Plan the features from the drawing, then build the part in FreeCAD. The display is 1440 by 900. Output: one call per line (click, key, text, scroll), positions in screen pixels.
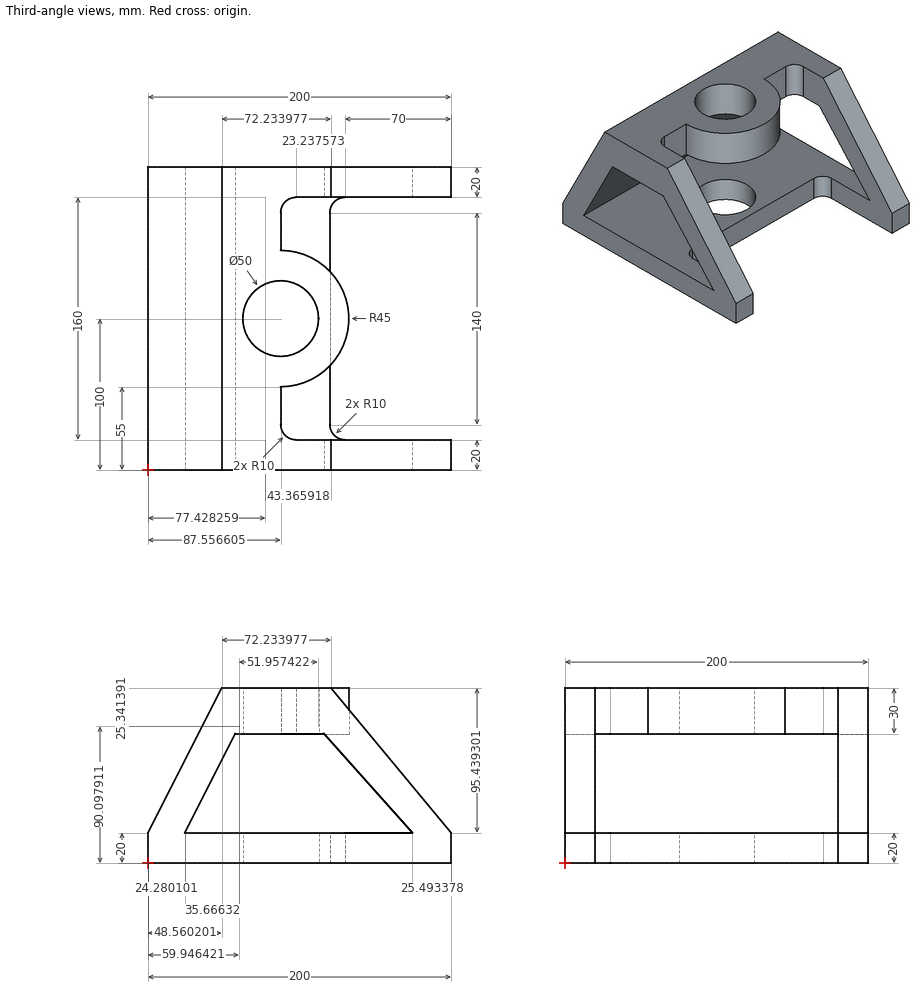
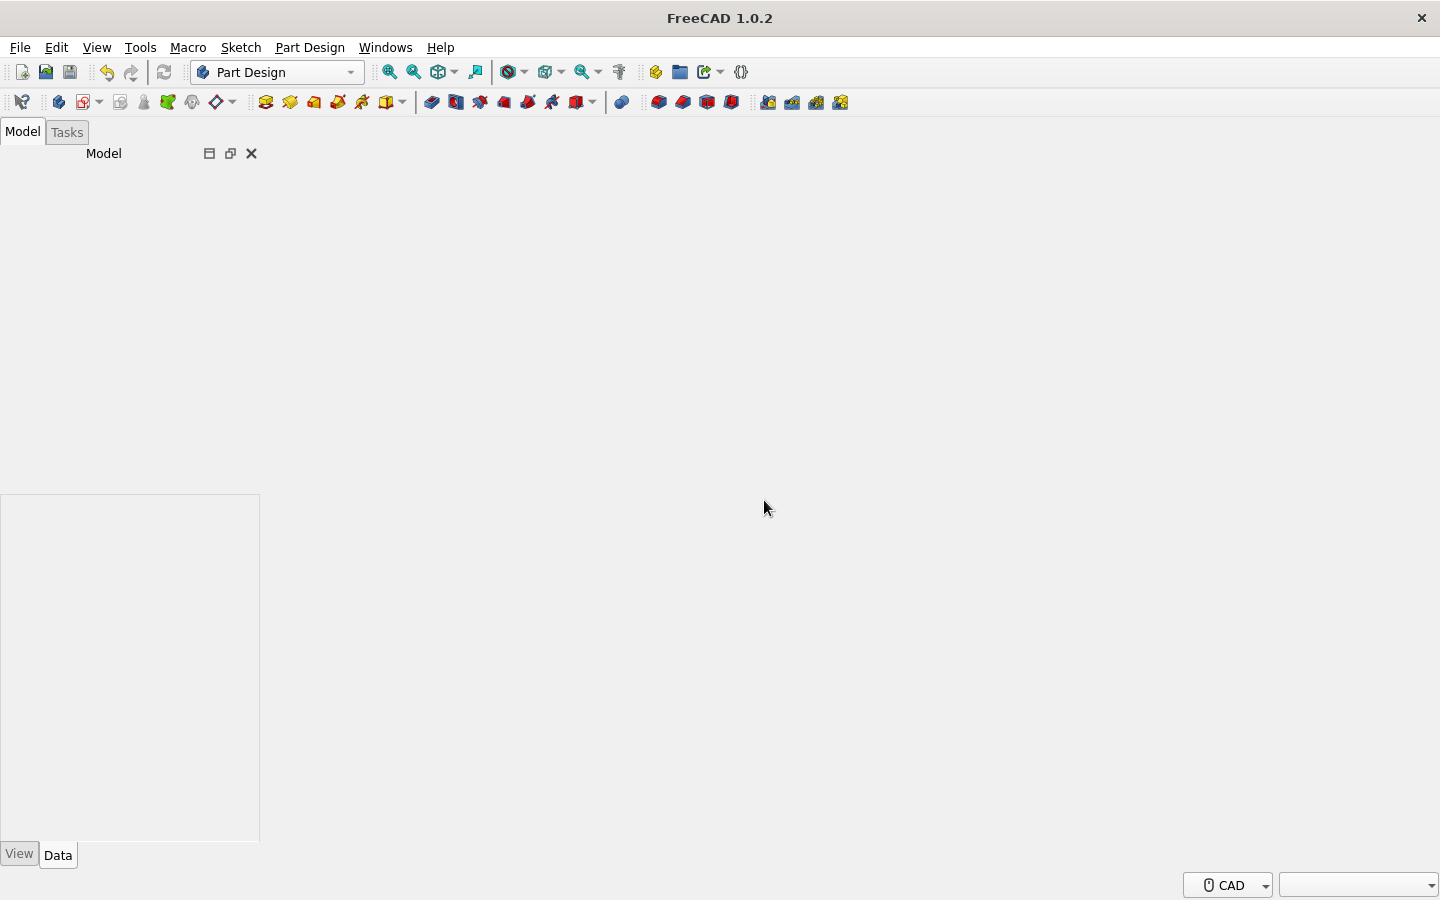
click(22, 72)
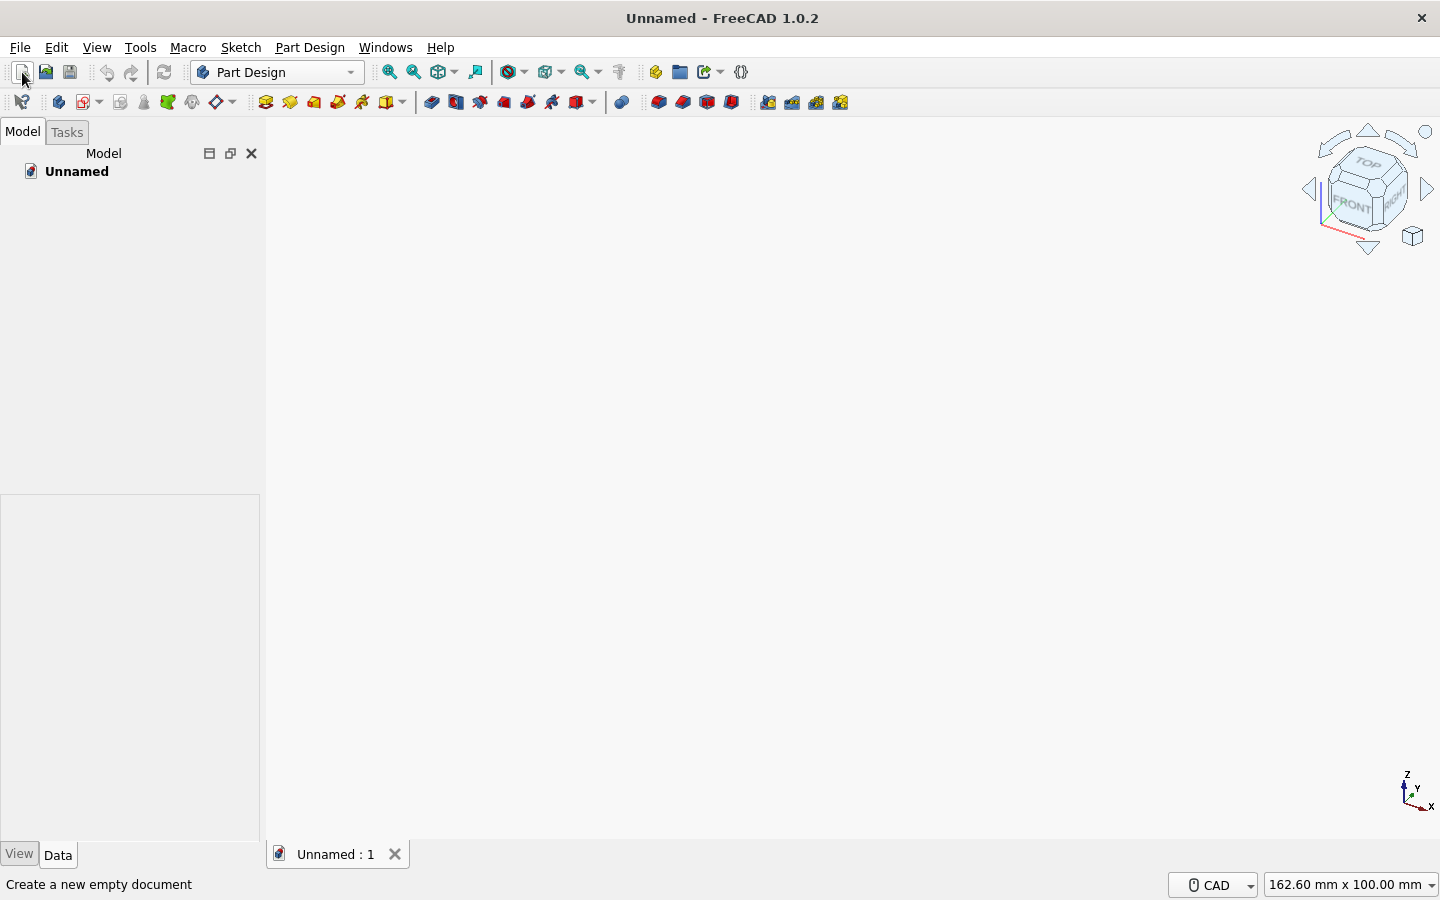
click(84, 102)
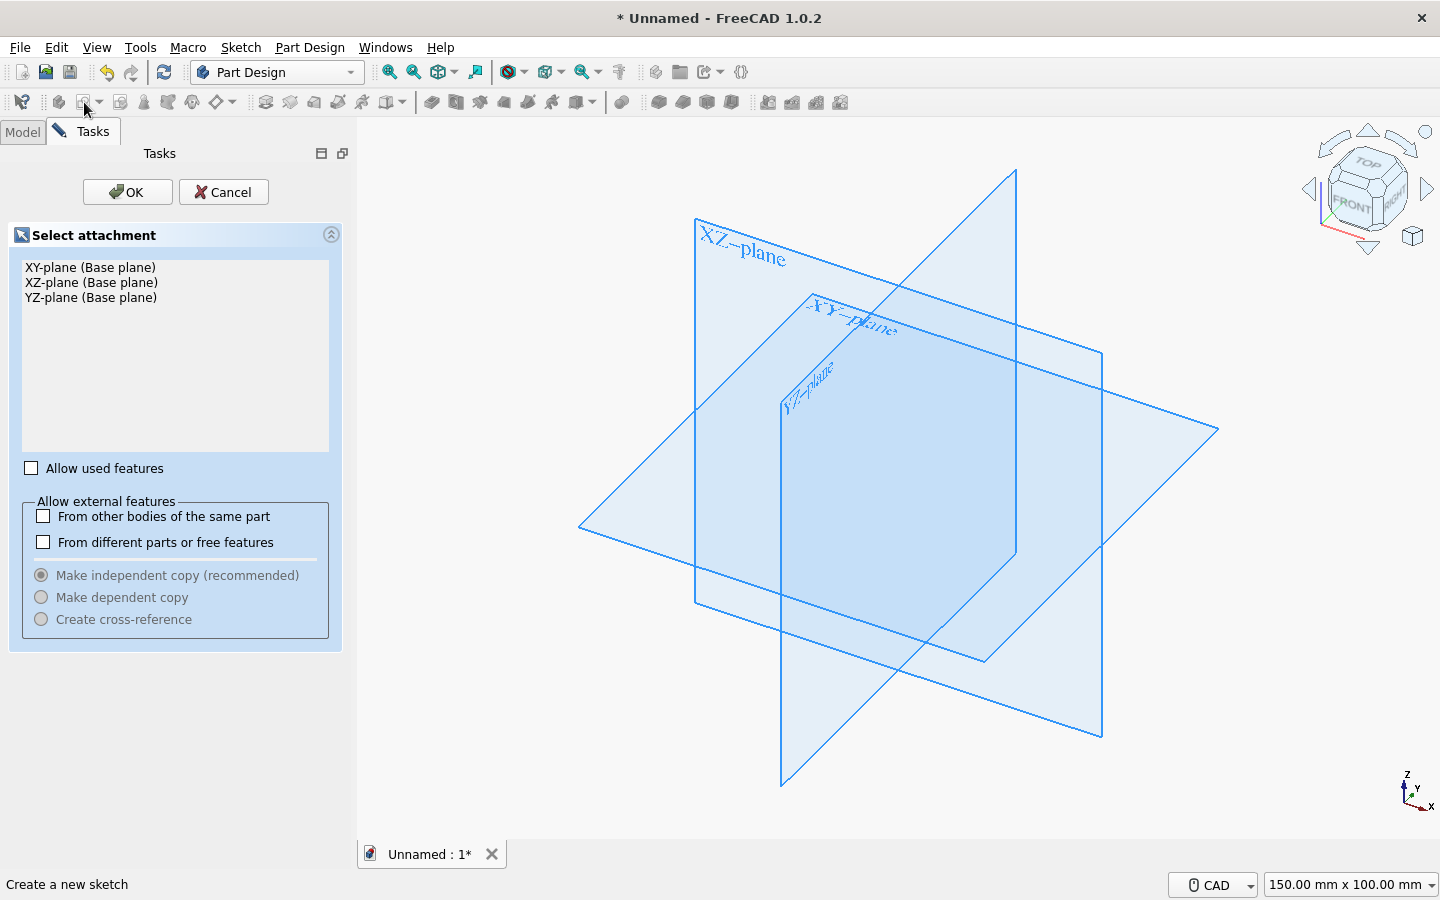
click(82, 268)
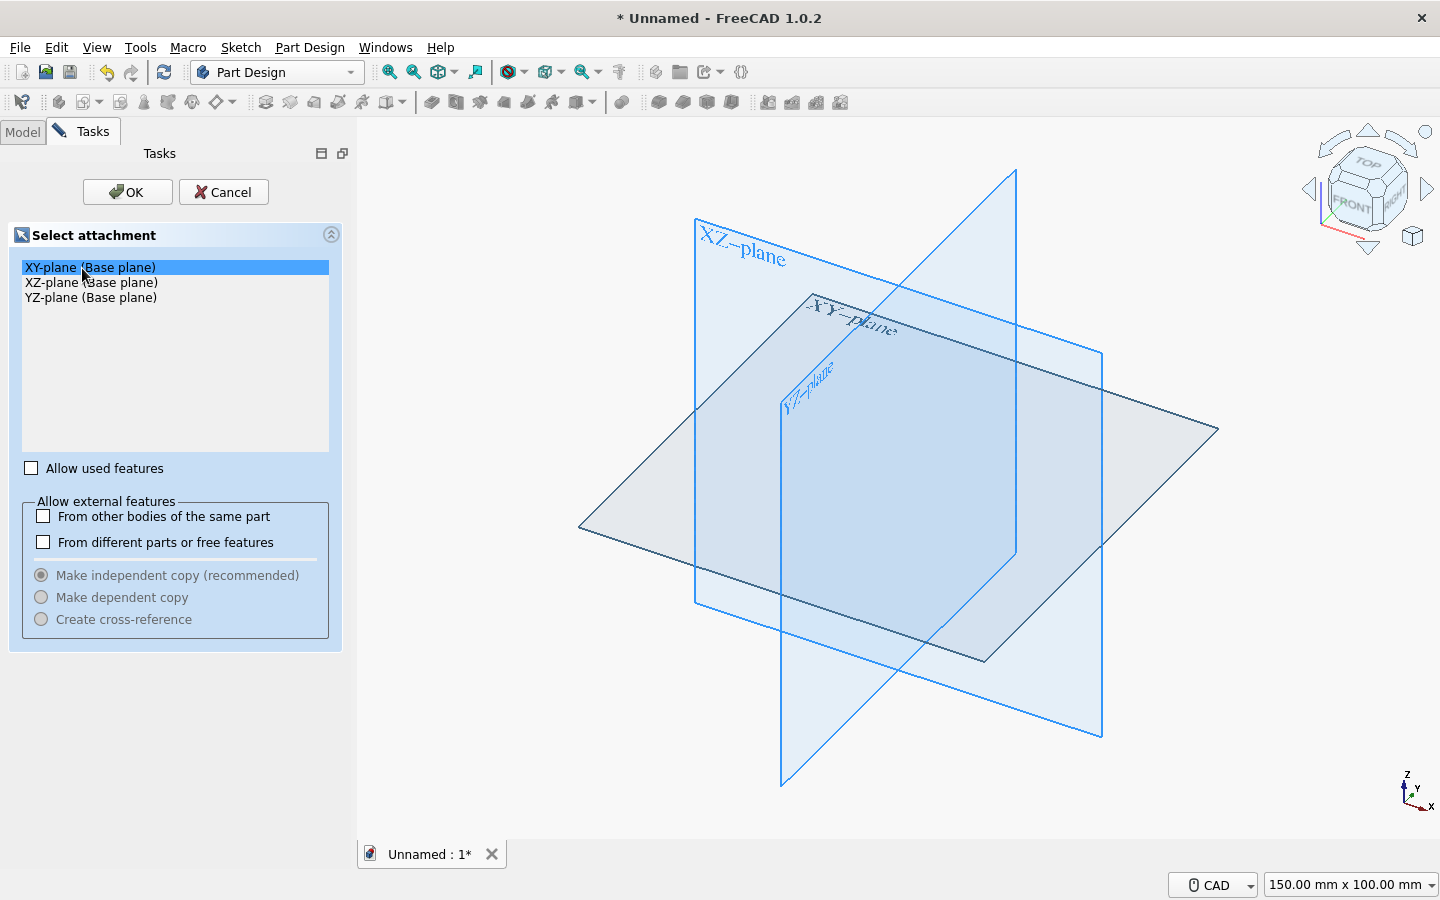
click(128, 192)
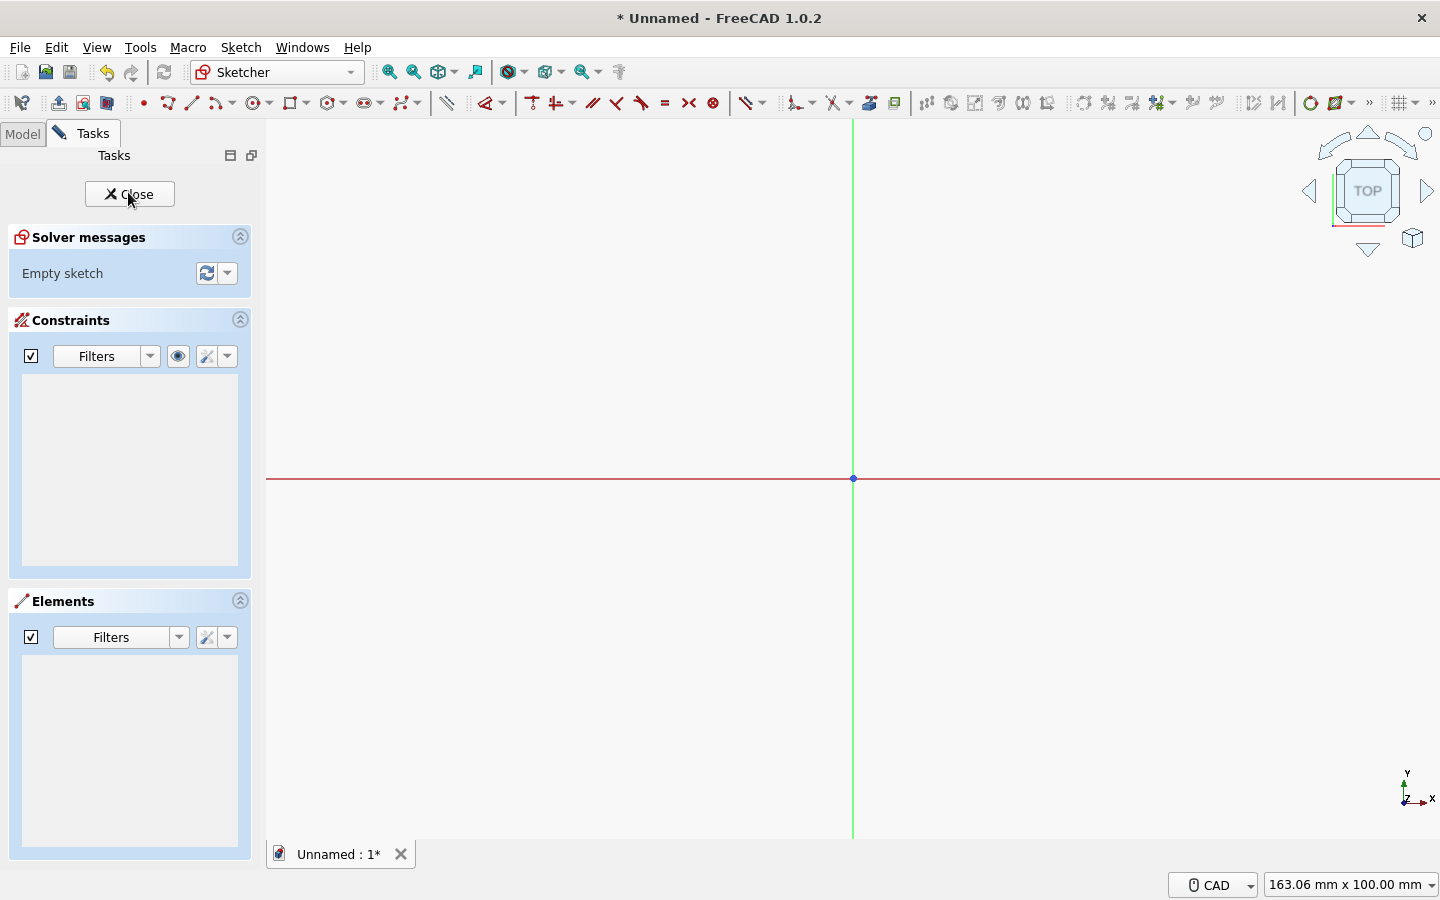
scroll(445, 789, down, 6)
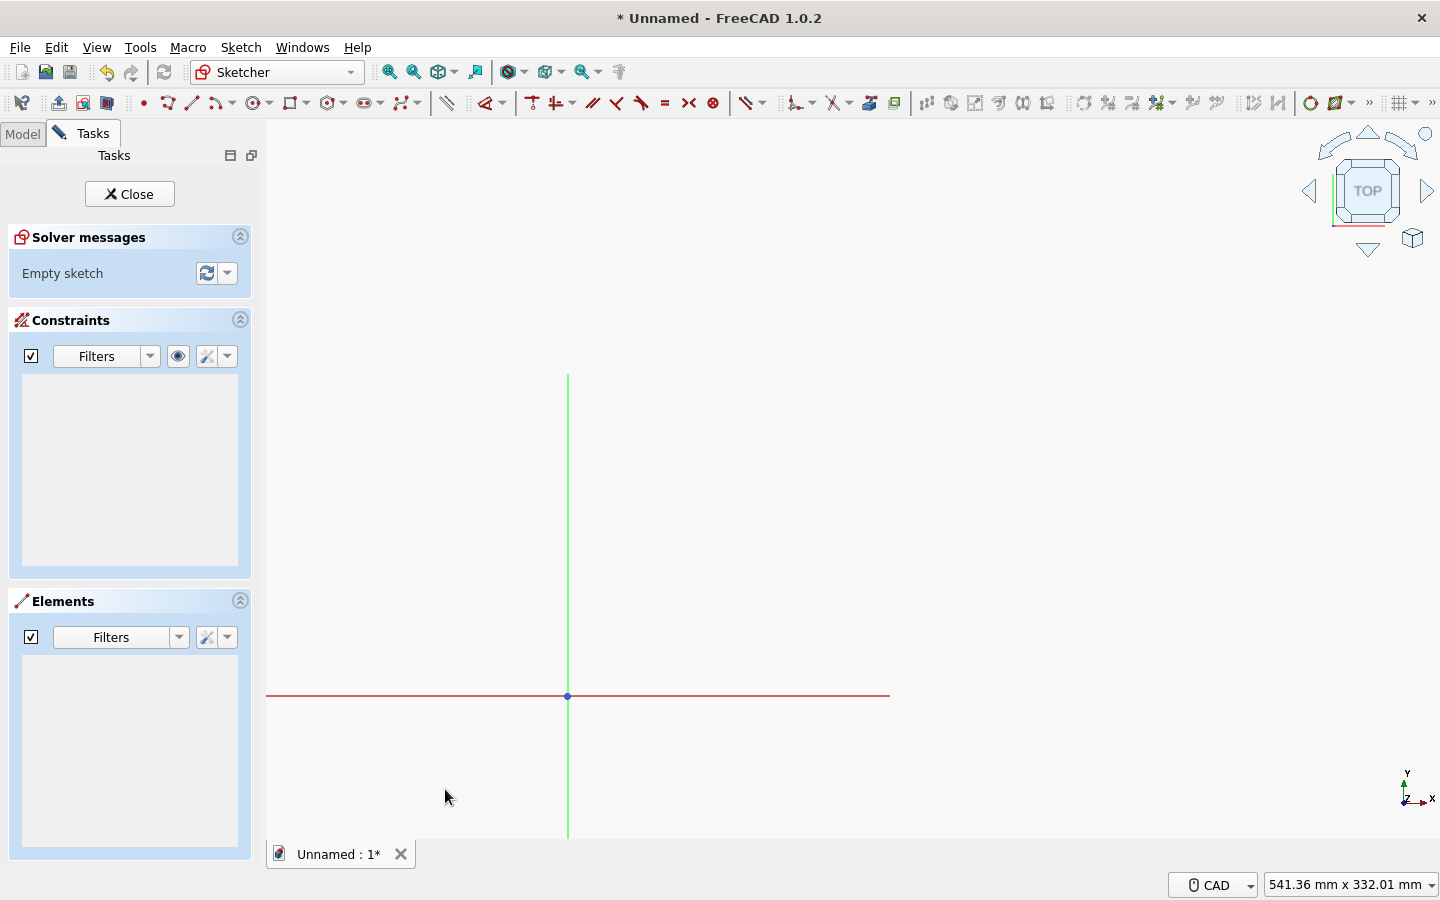
click(192, 104)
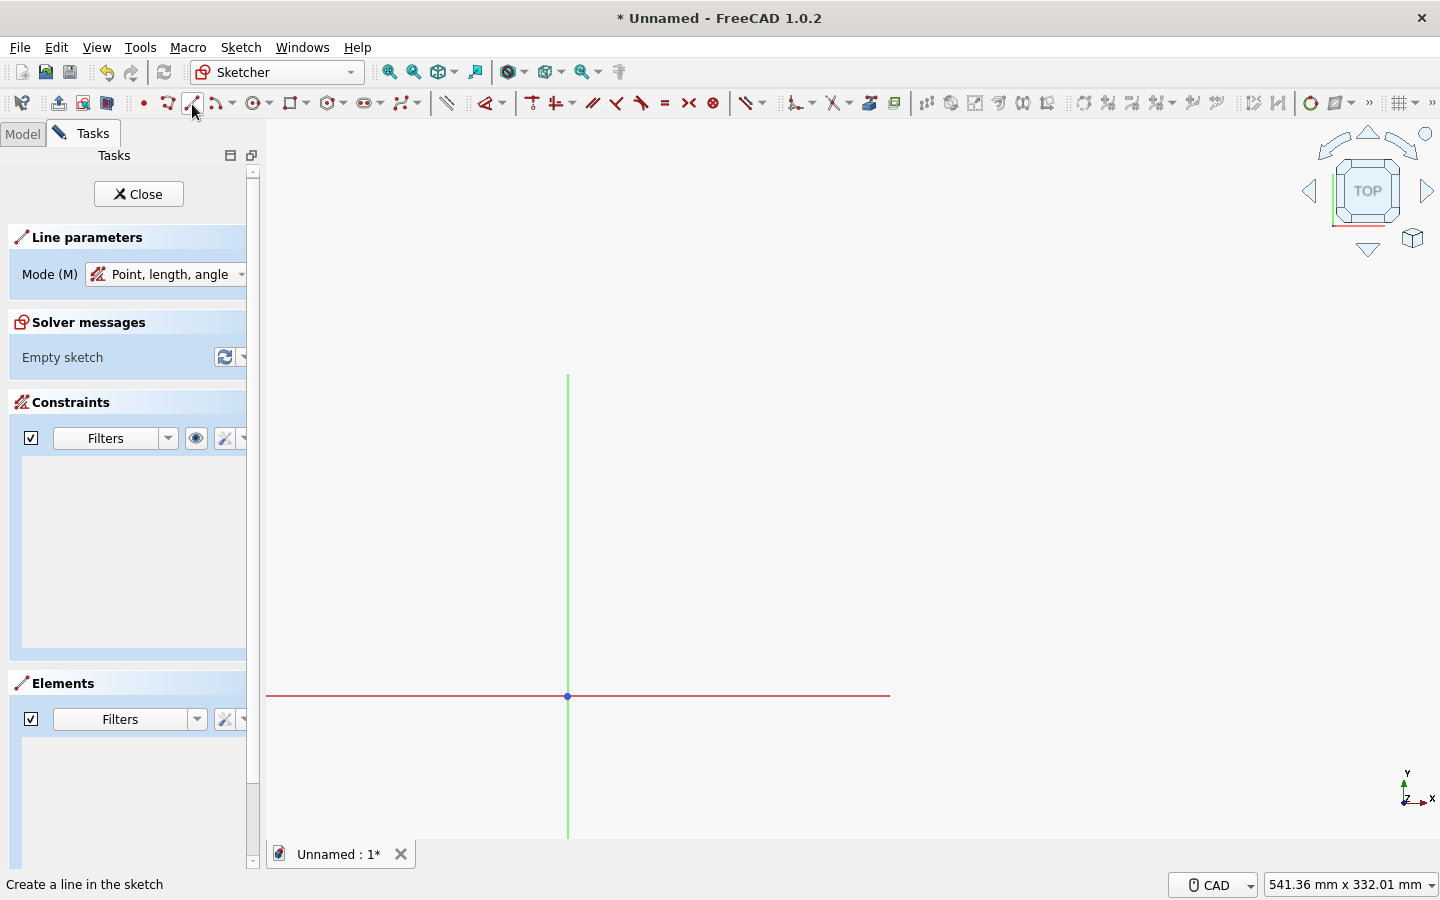
click(828, 631)
click(828, 328)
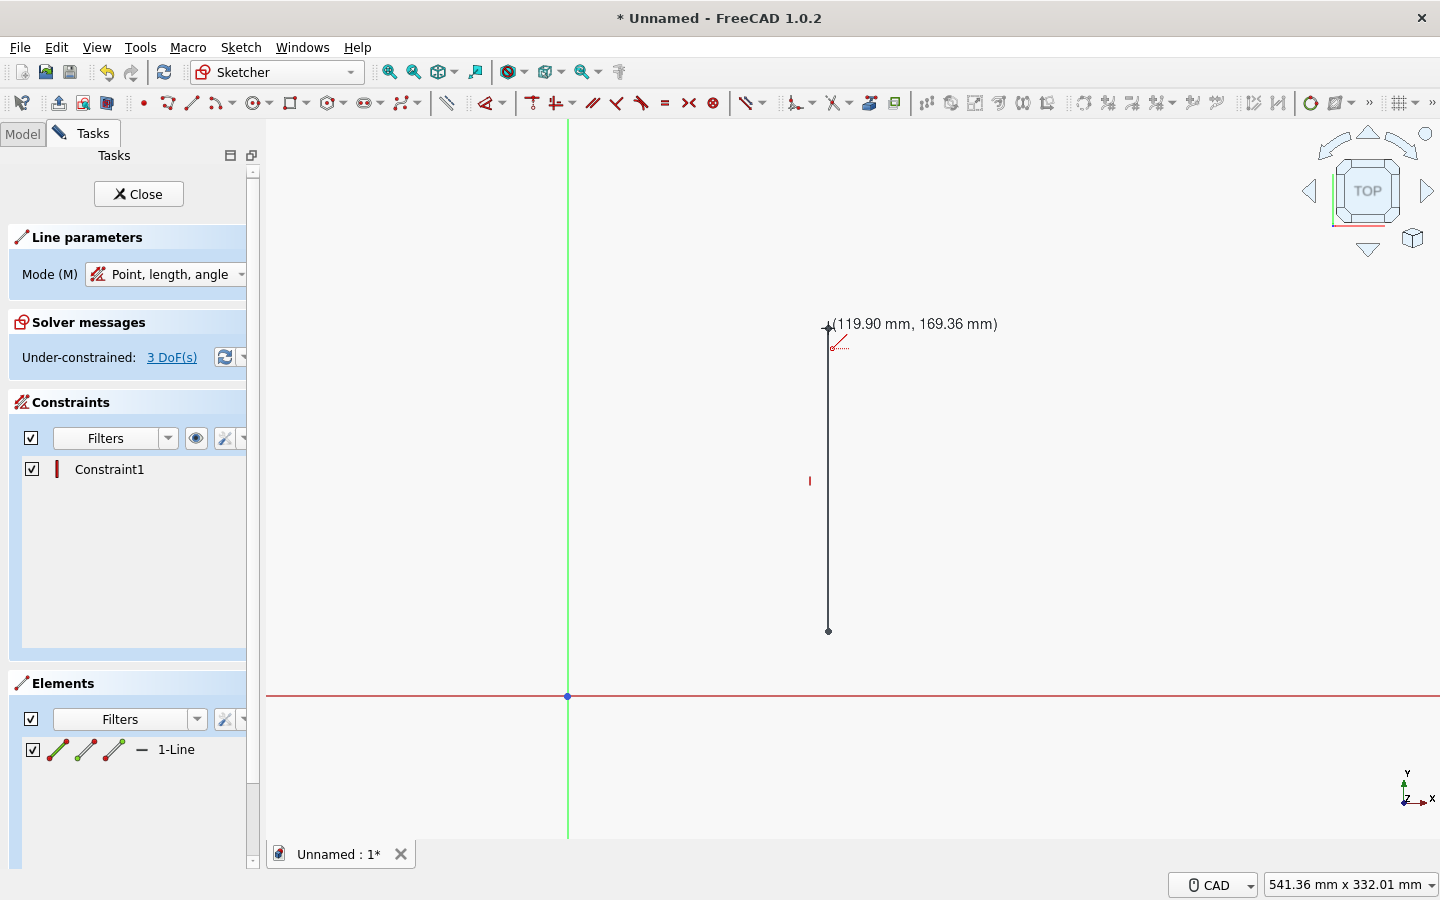
click(168, 104)